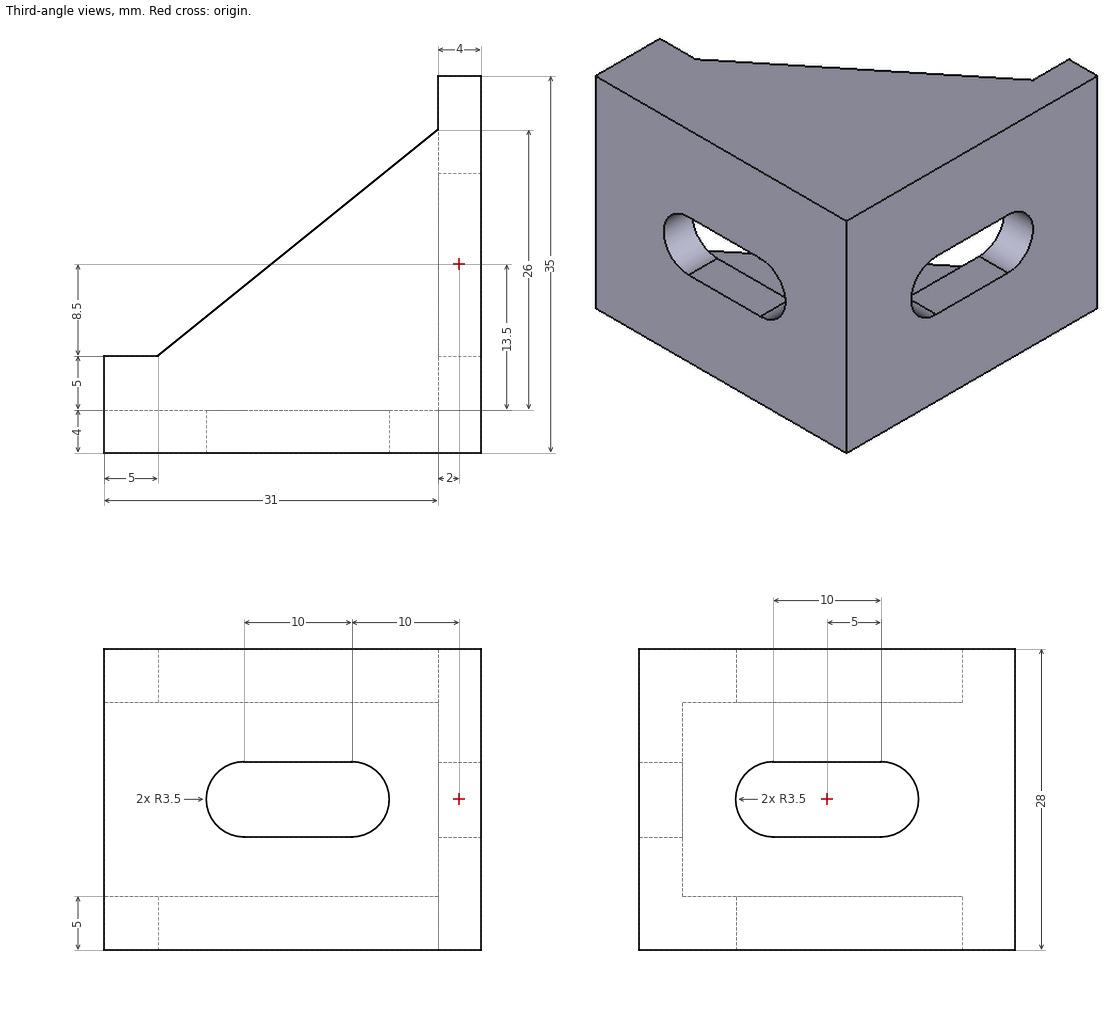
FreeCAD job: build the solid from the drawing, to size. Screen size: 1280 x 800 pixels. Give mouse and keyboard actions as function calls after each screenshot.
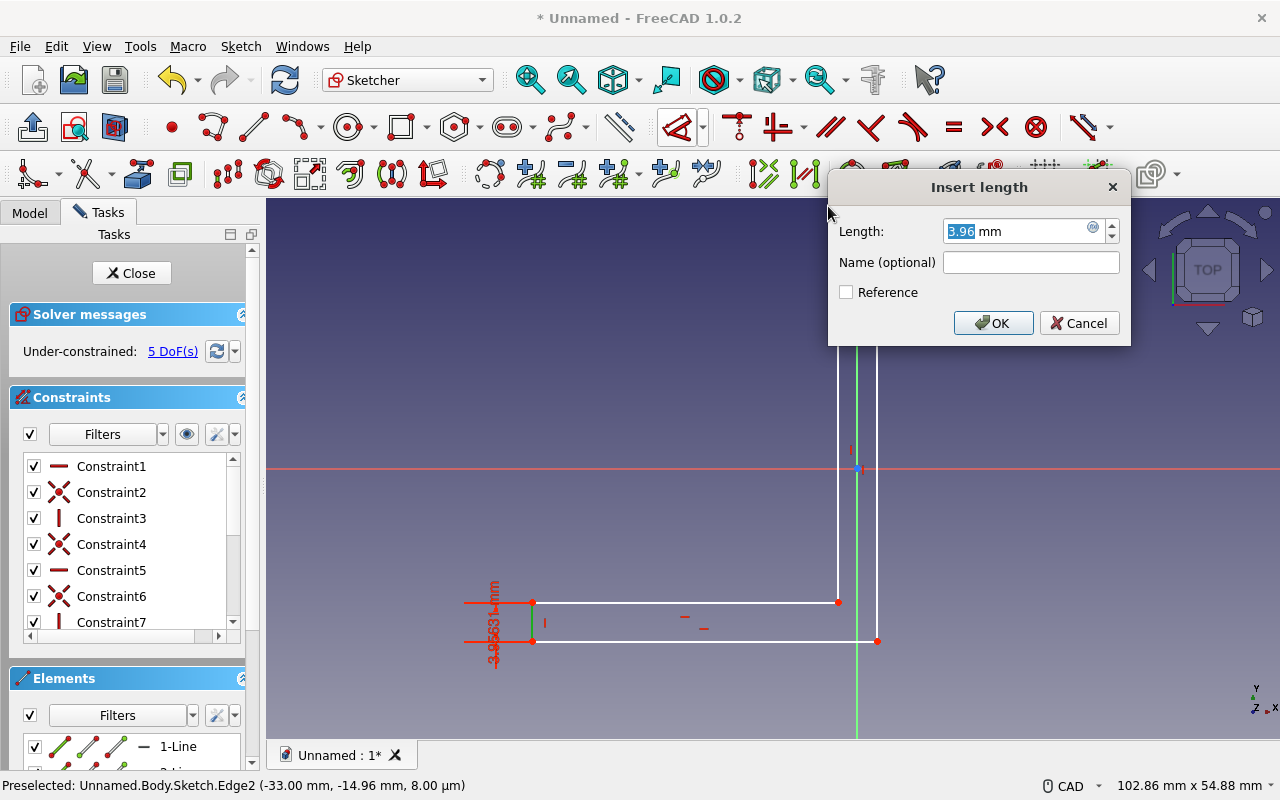
text(4)
key(Return)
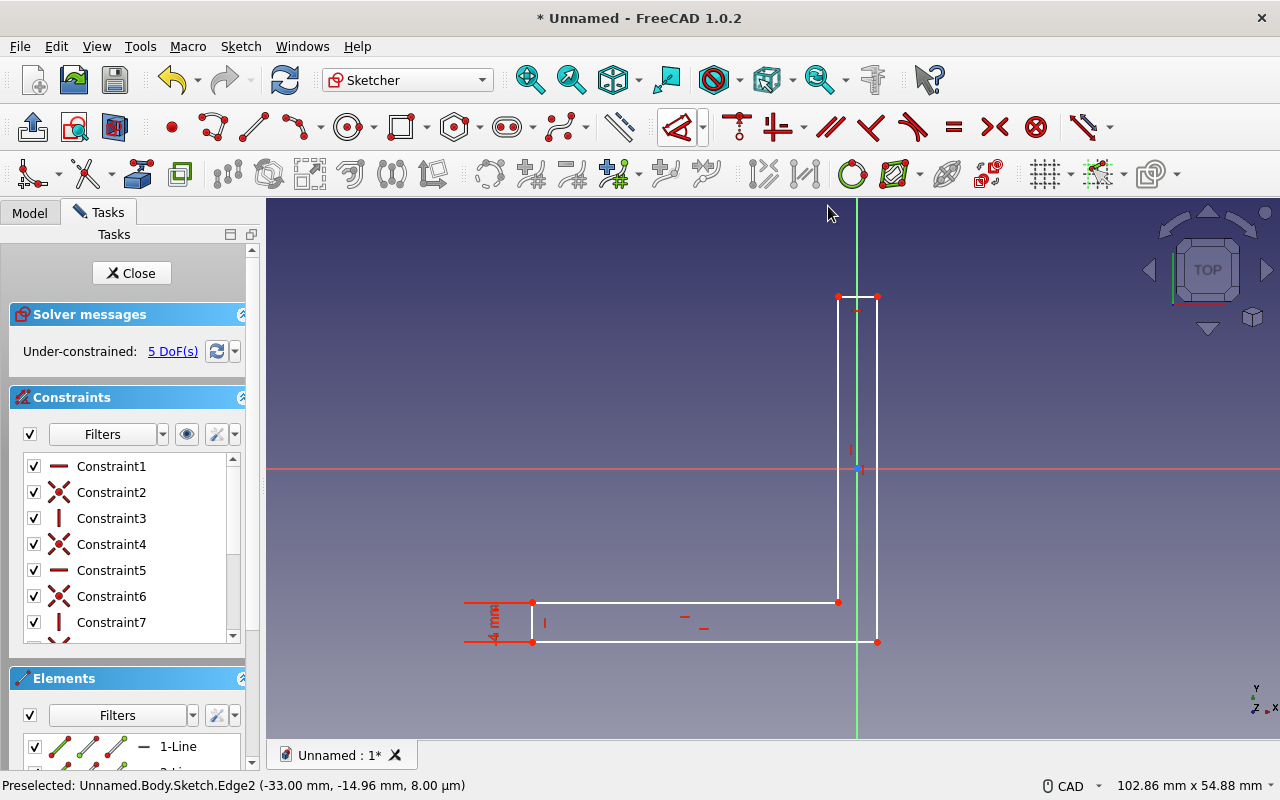
click(854, 297)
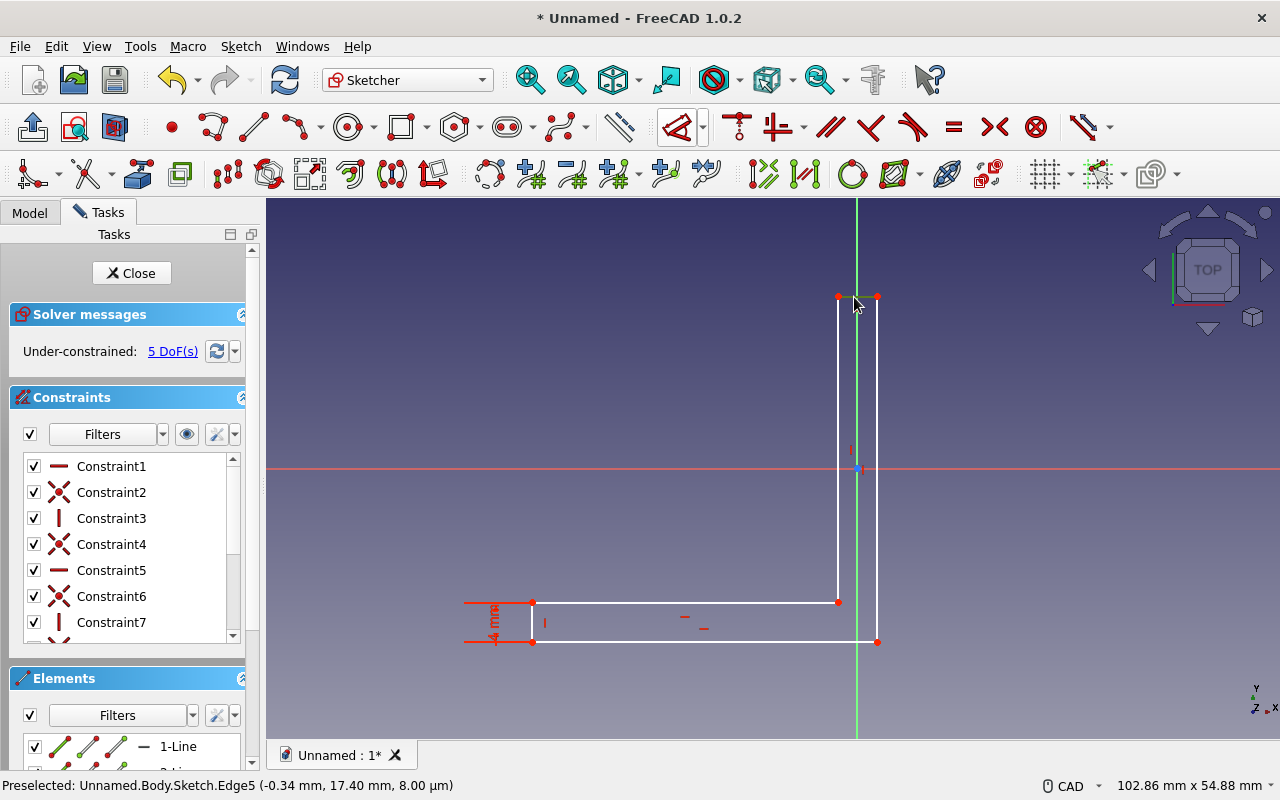
click(702, 128)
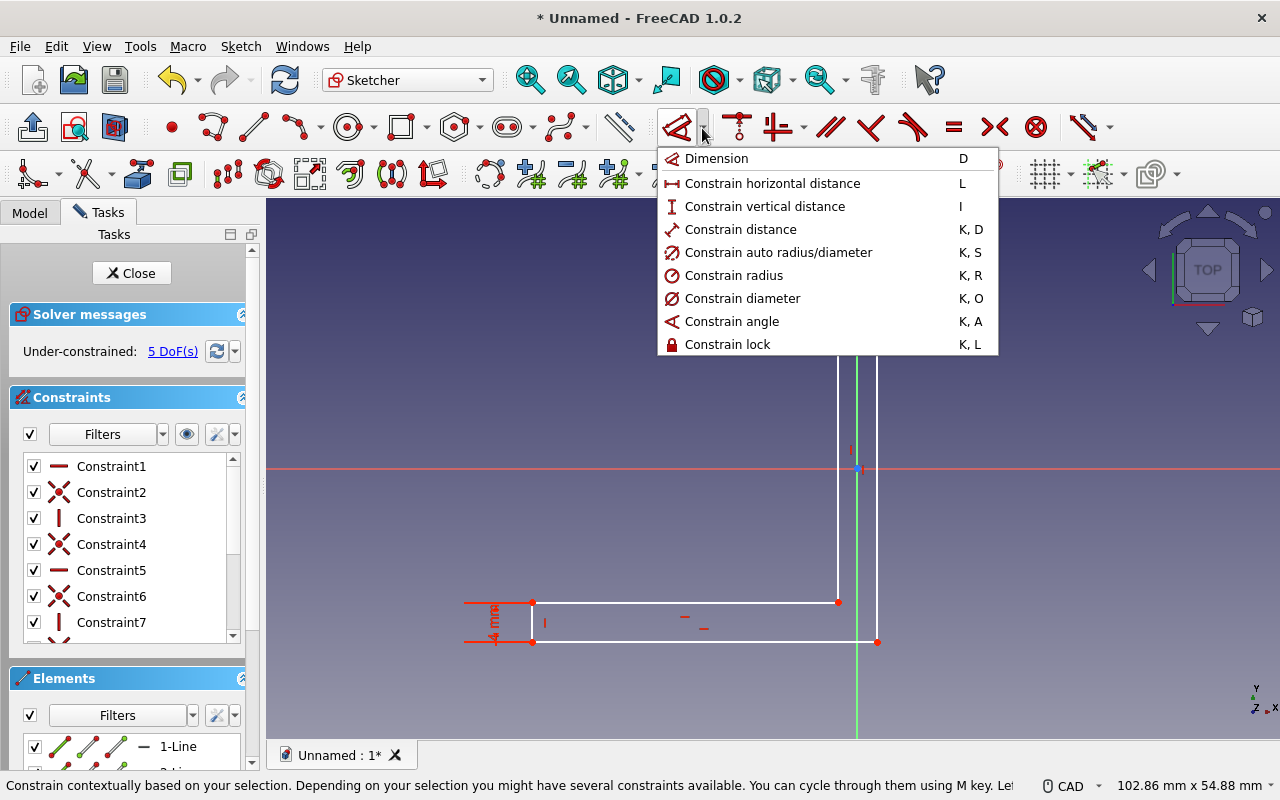
click(828, 184)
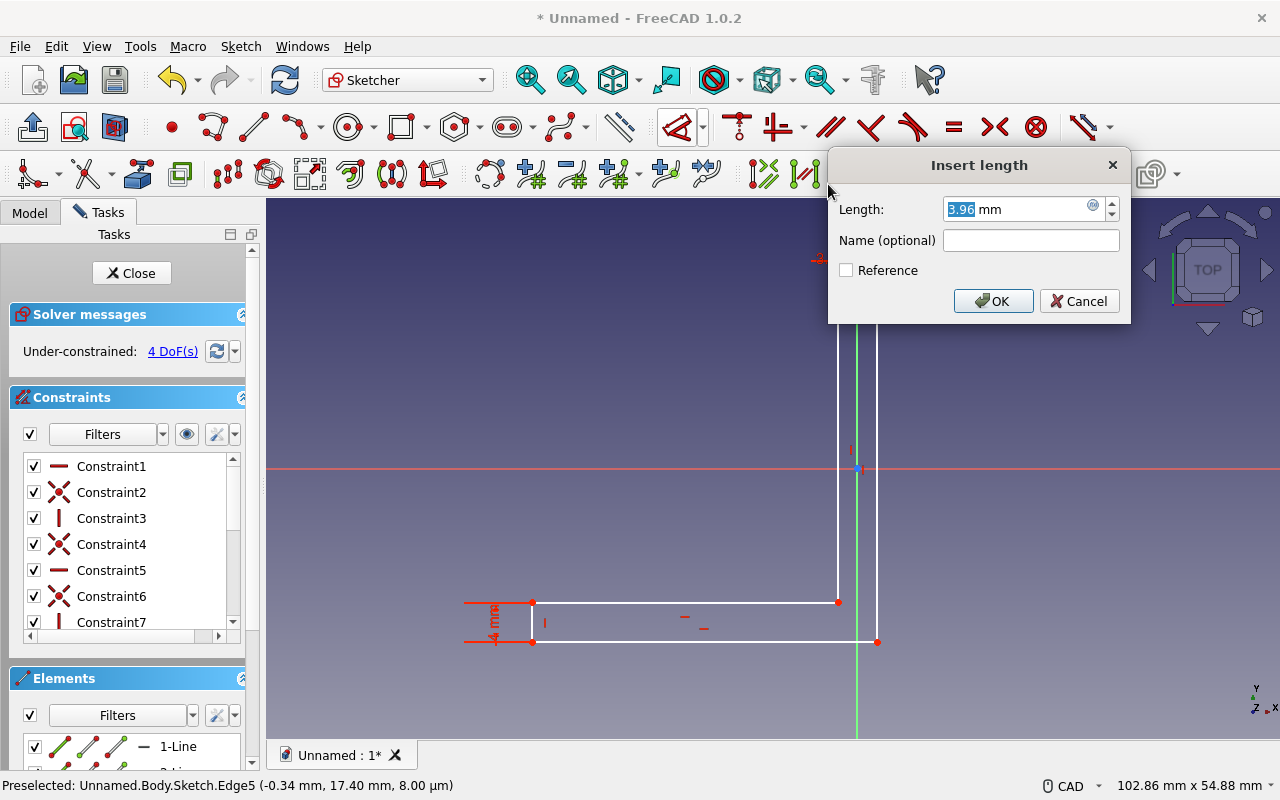
text(4)
key(Return)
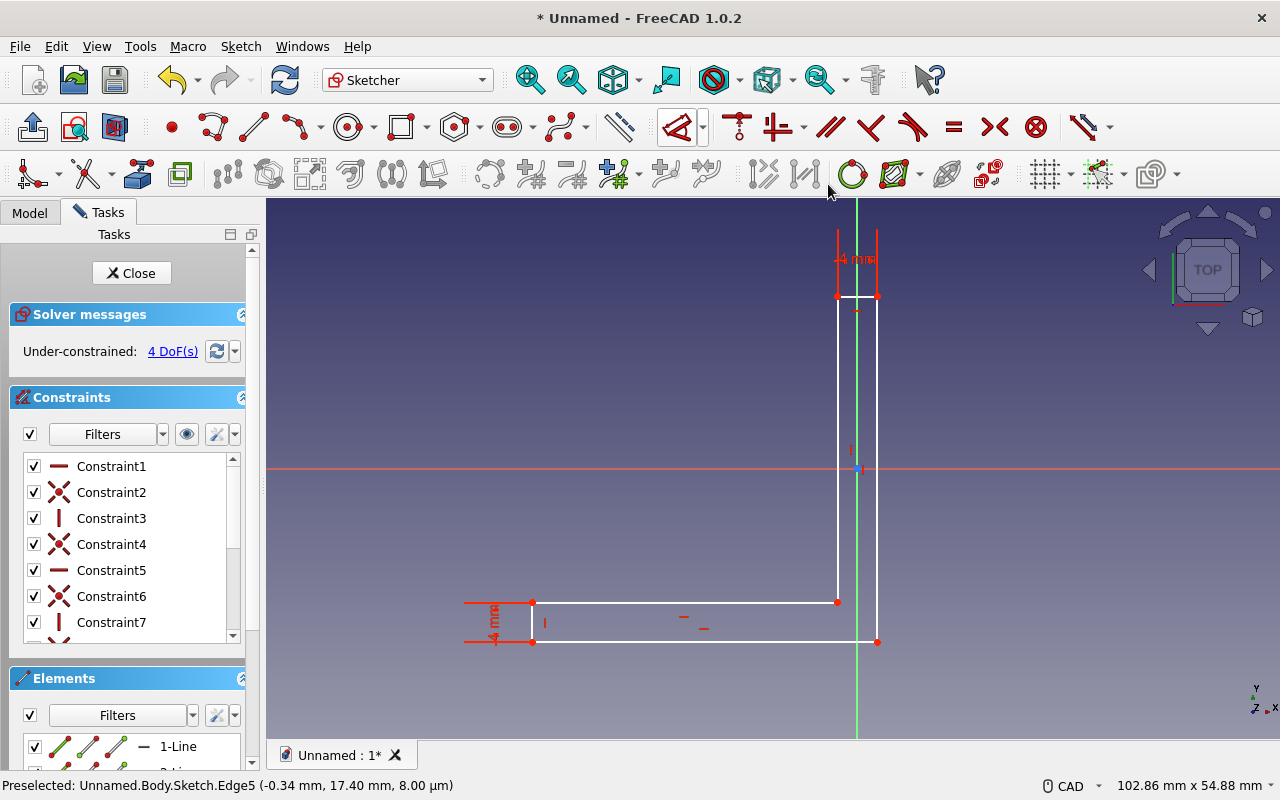
click(746, 603)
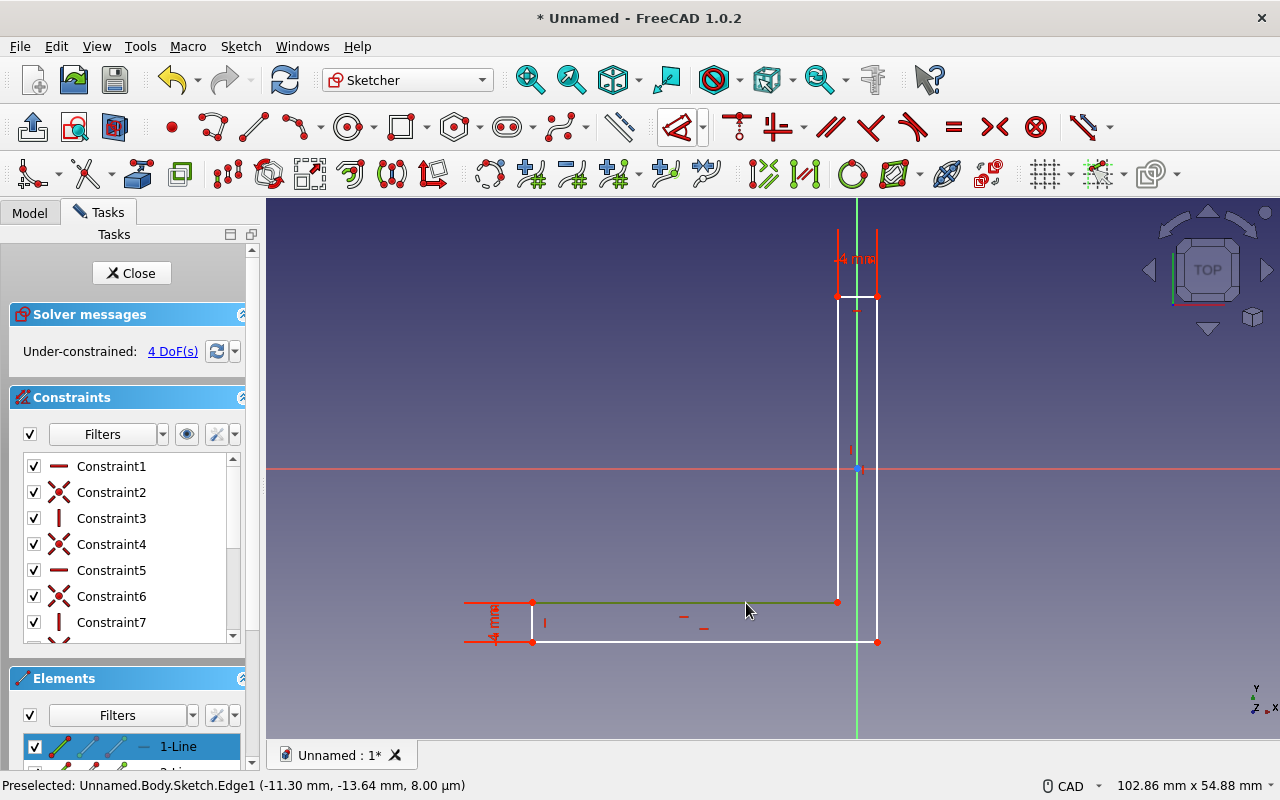
click(702, 128)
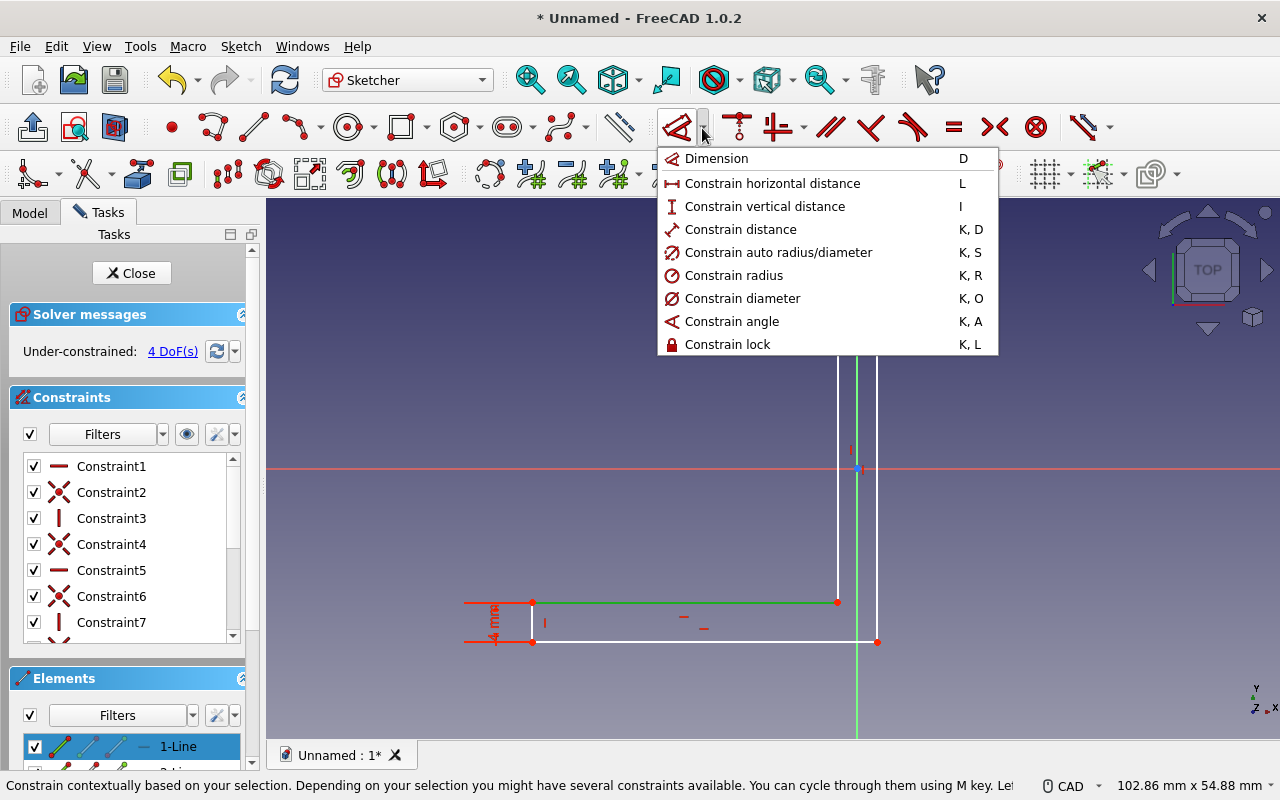
click(828, 184)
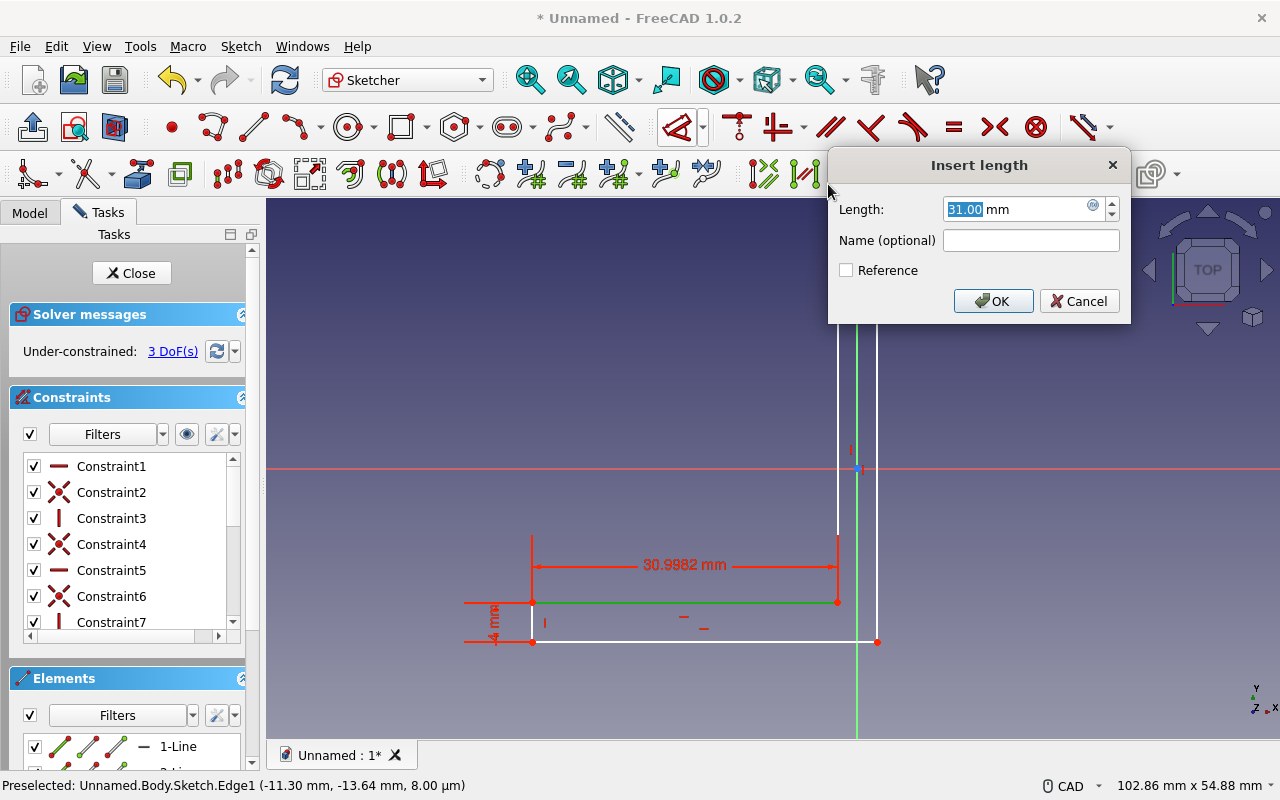
text(31)
key(Return)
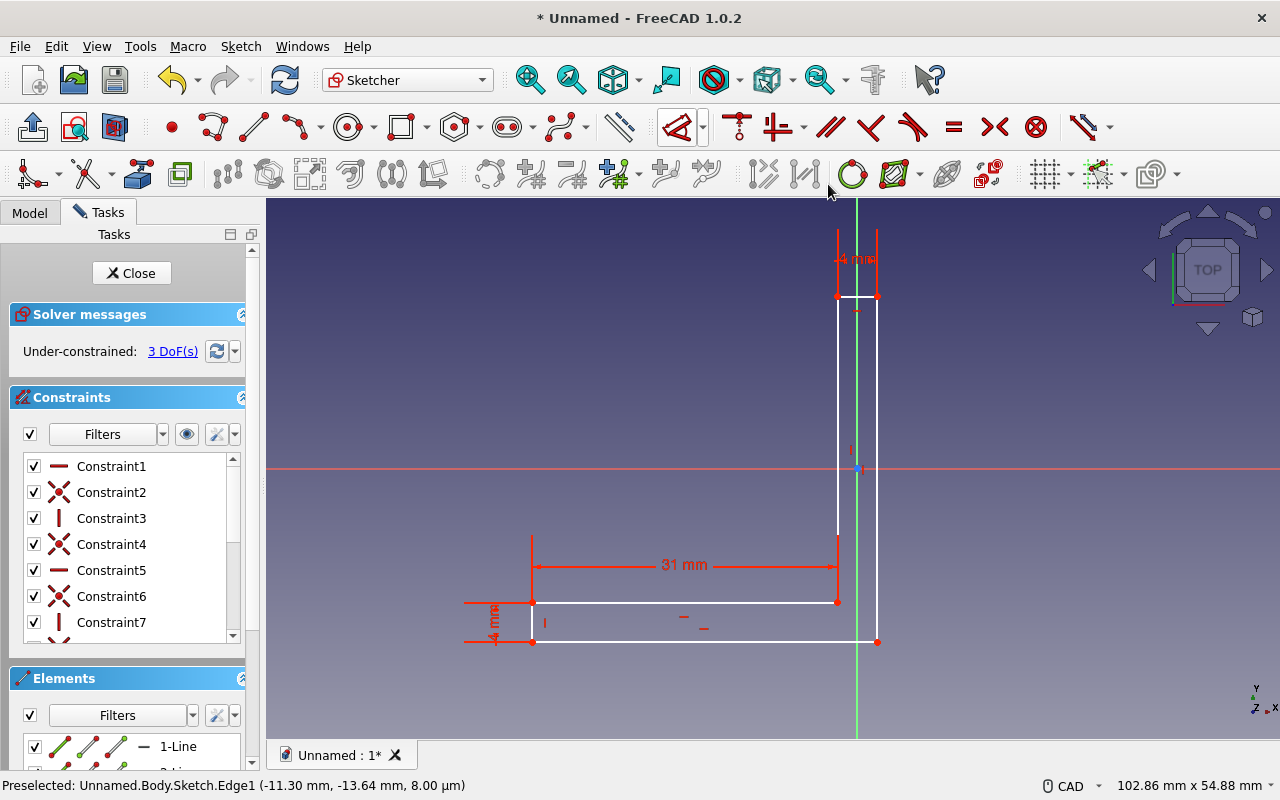
click(877, 539)